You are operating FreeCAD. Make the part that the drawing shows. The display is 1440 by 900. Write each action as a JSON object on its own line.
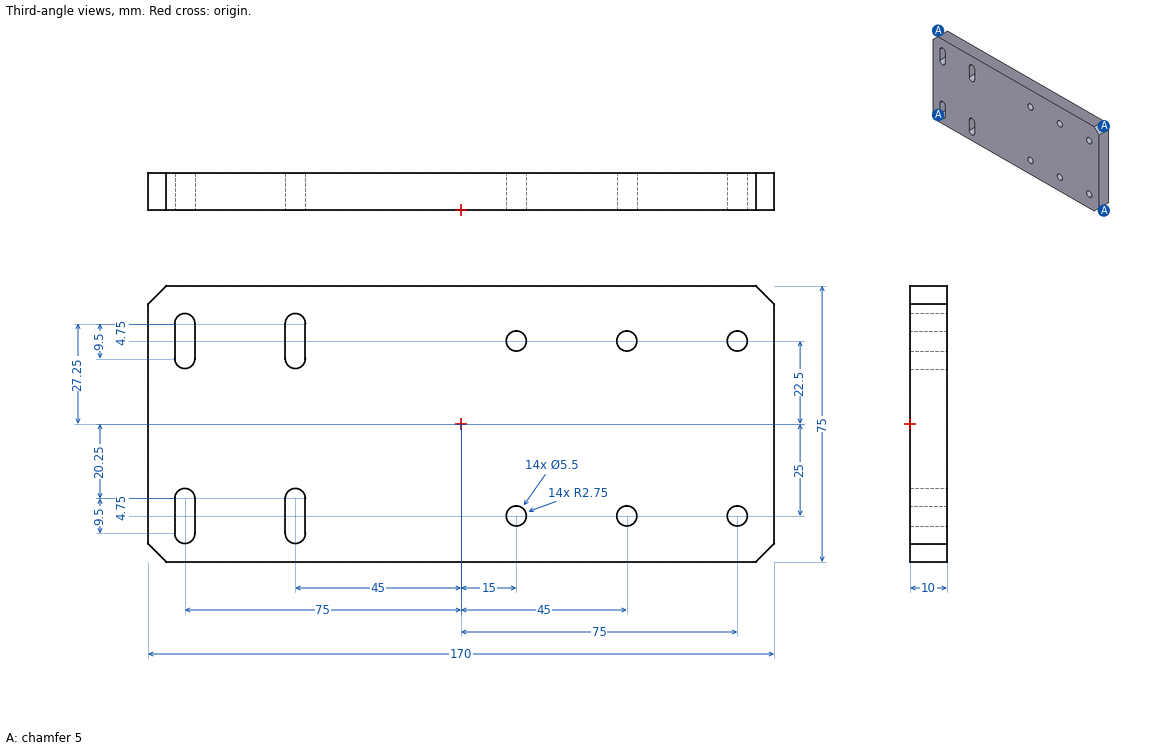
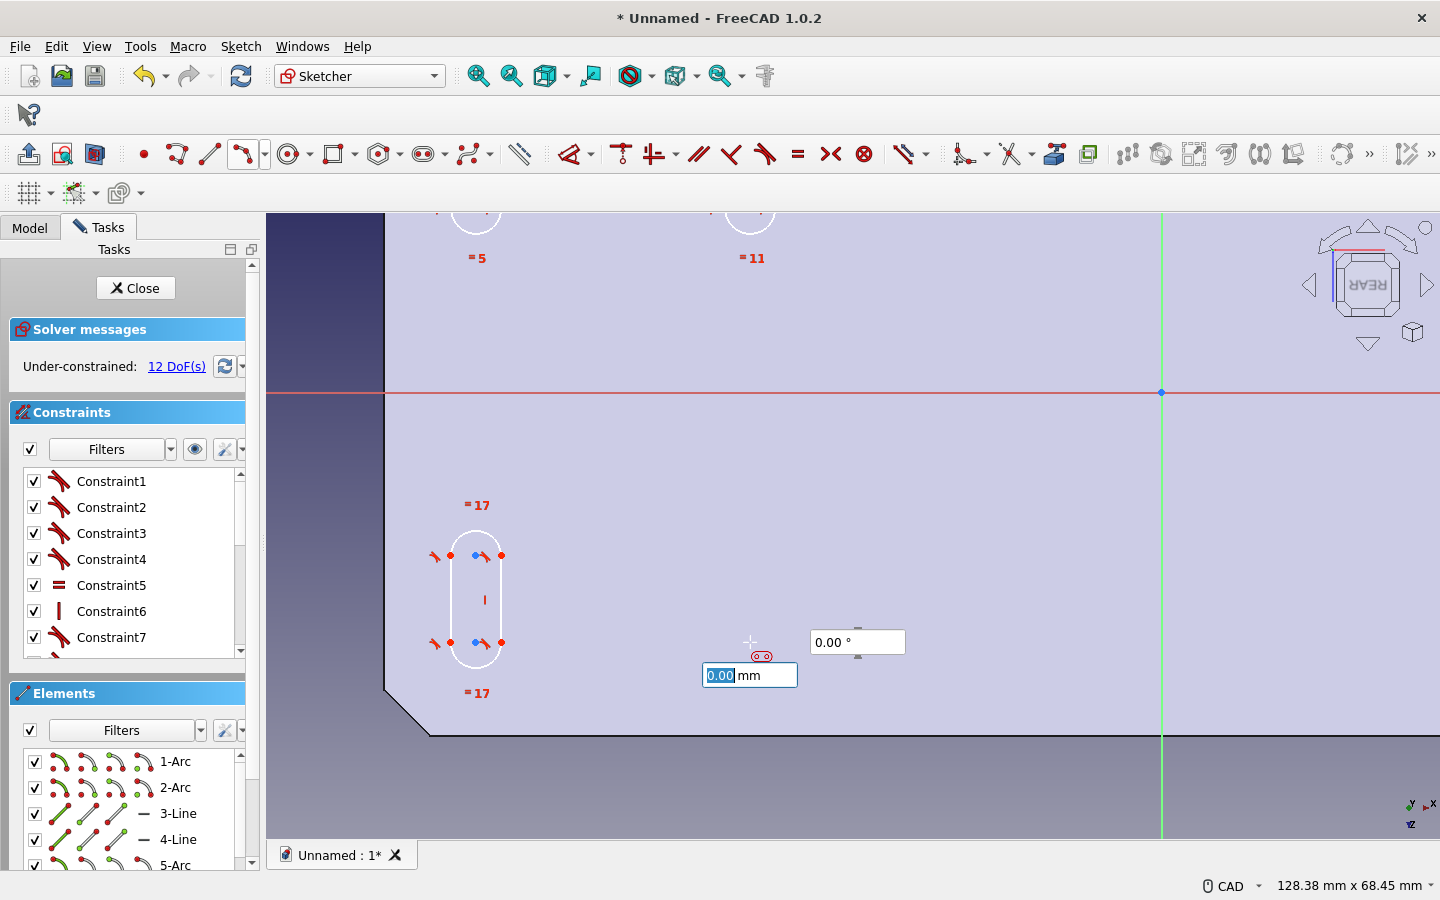
{"action": "left_click", "coordinate": [750, 555]}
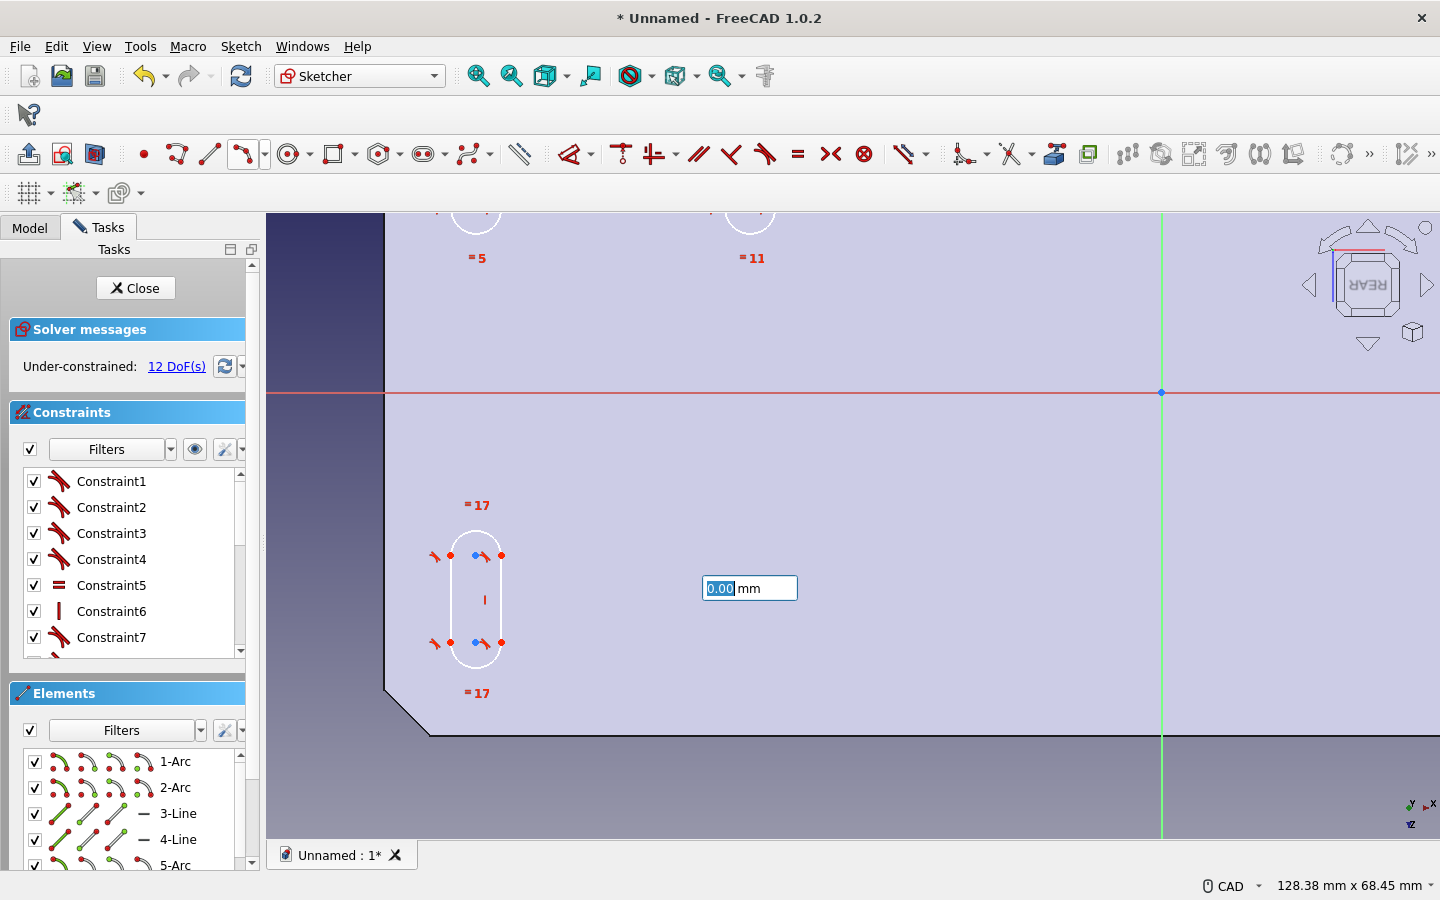
{"action": "left_click", "coordinate": [775, 599]}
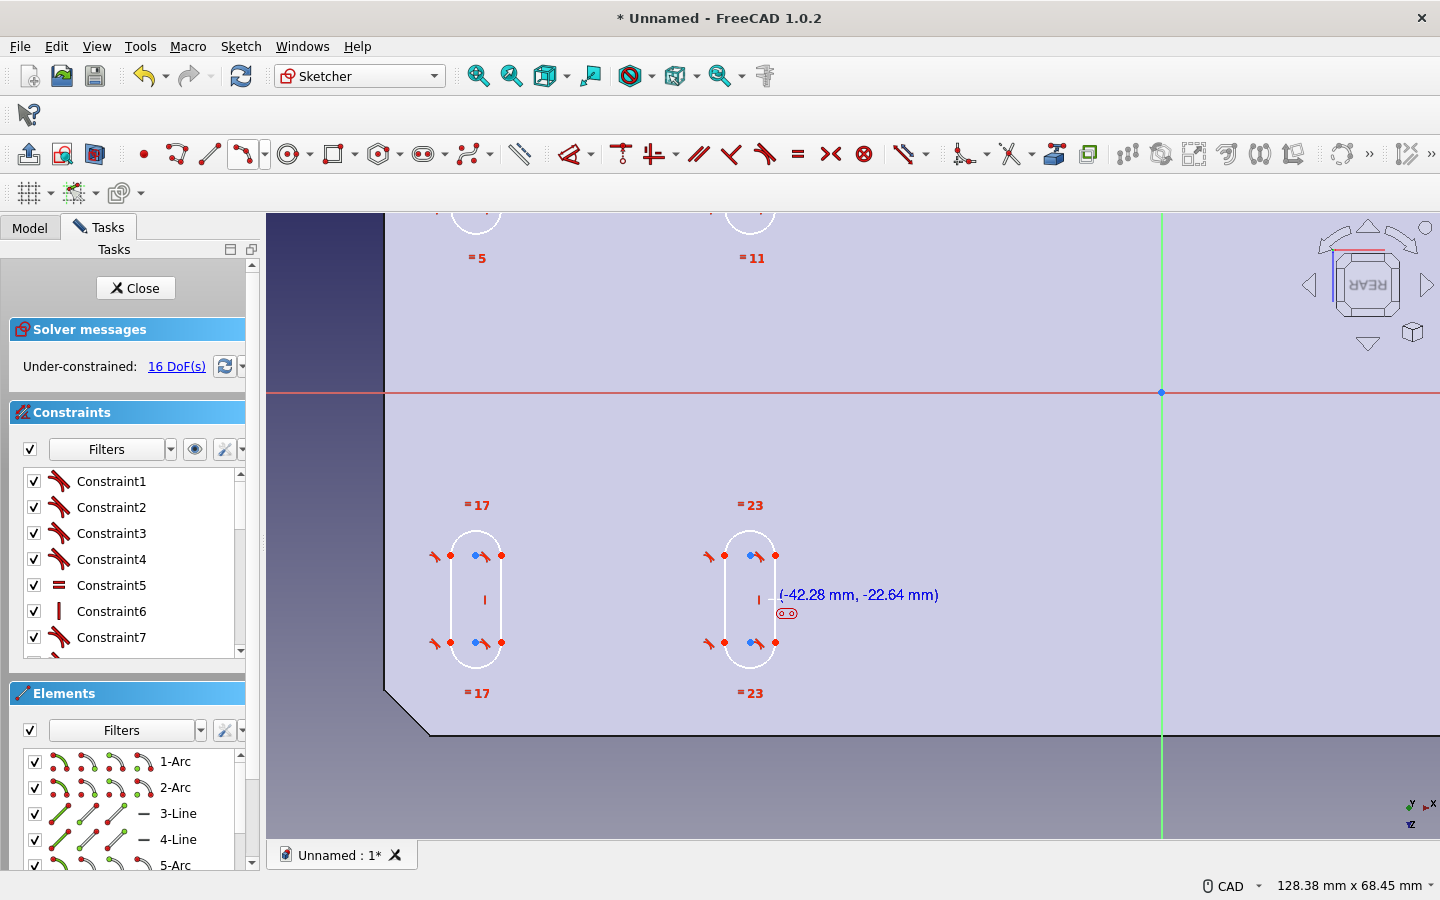
{"action": "key", "text": "g c"}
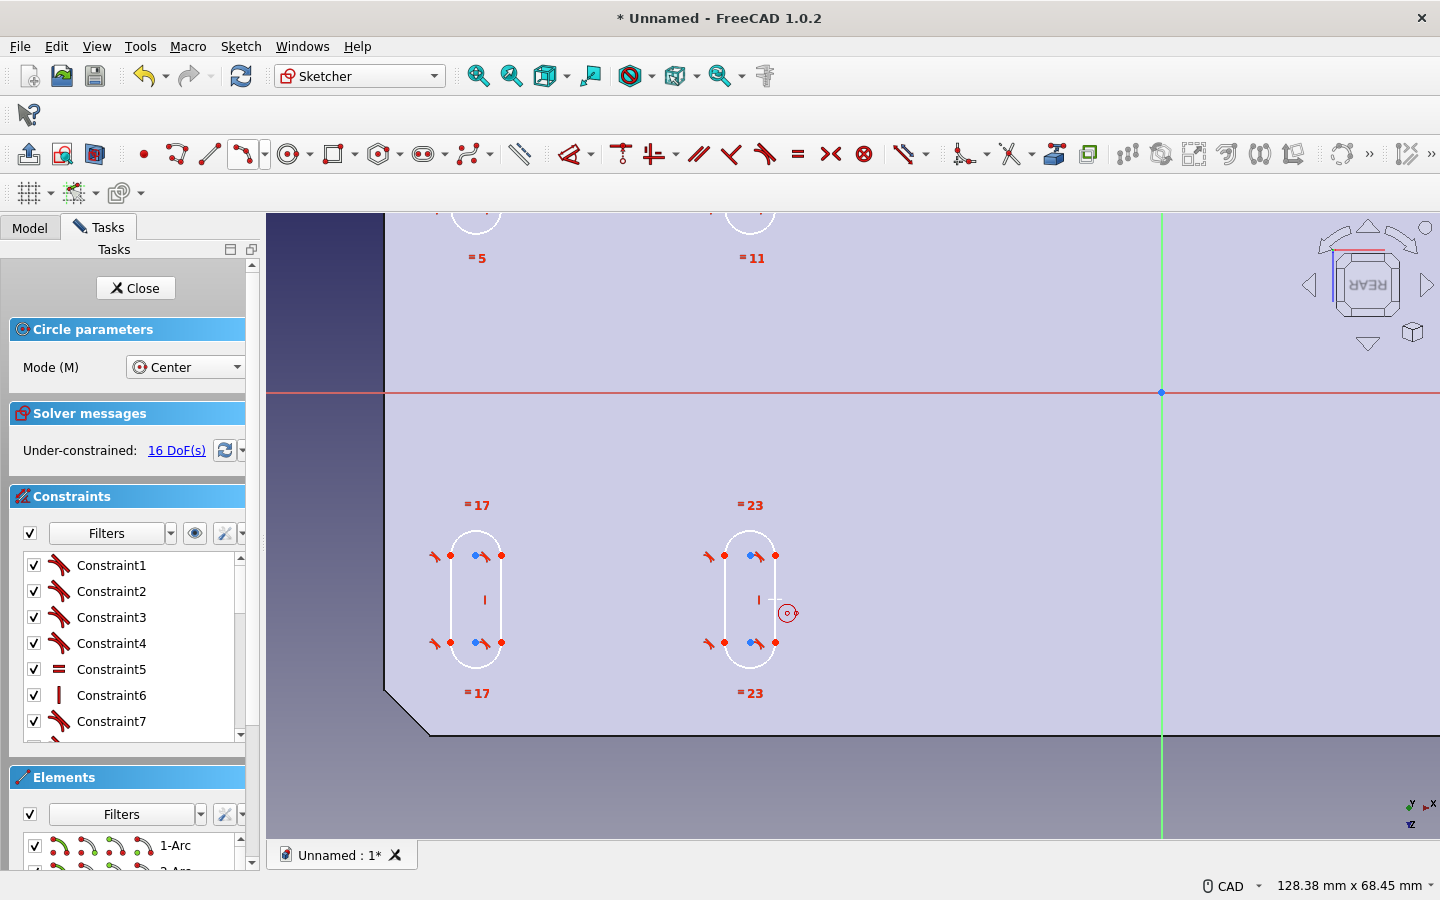
{"action": "scroll", "coordinate": [477, 644], "scroll_direction": "down", "scroll_amount": 4}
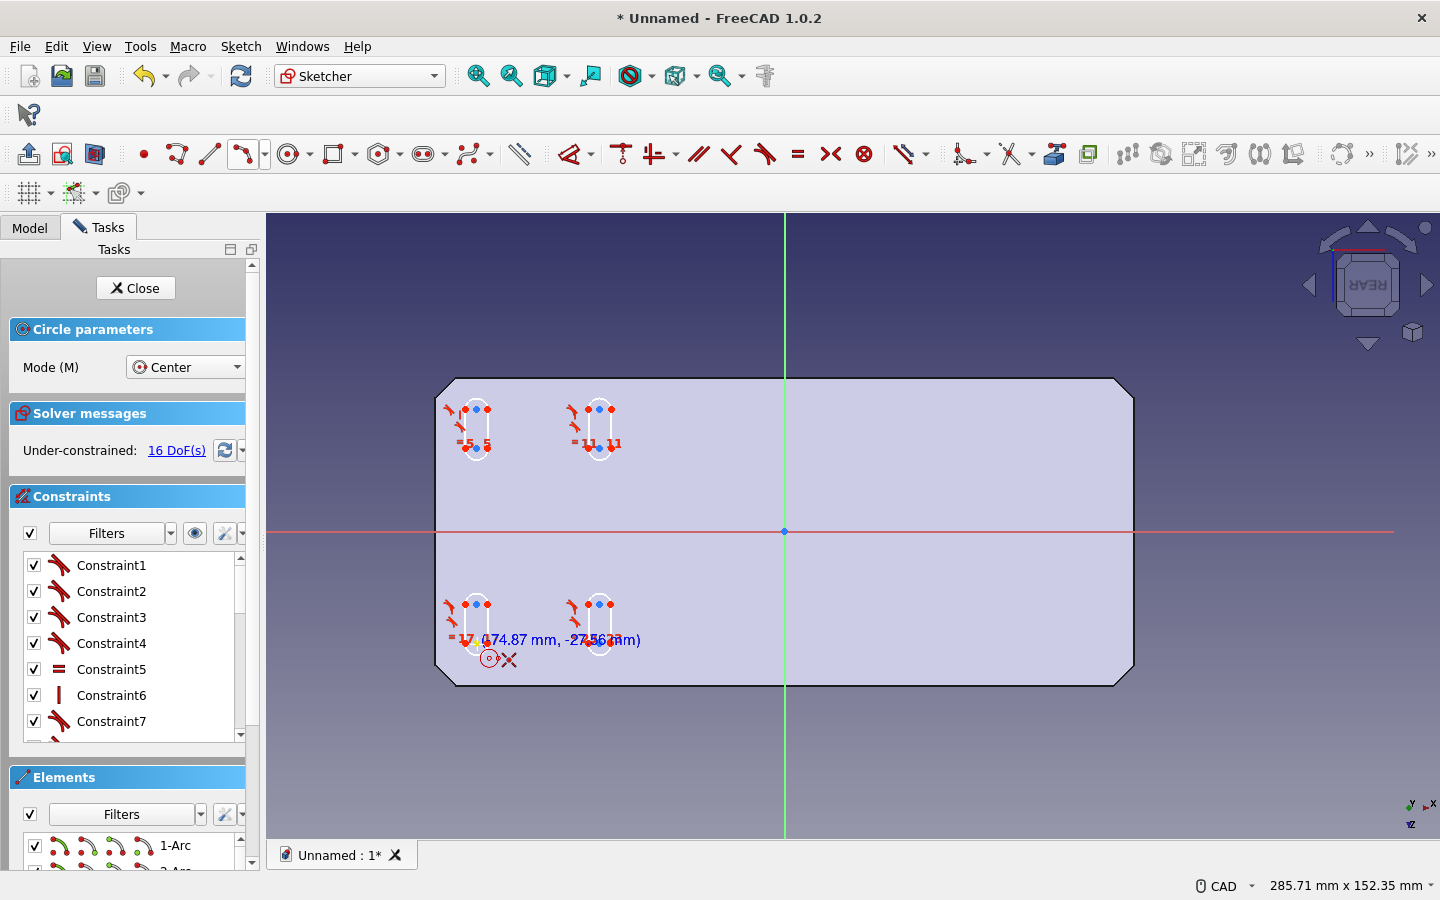
{"action": "scroll", "coordinate": [846, 429], "scroll_direction": "up", "scroll_amount": 4}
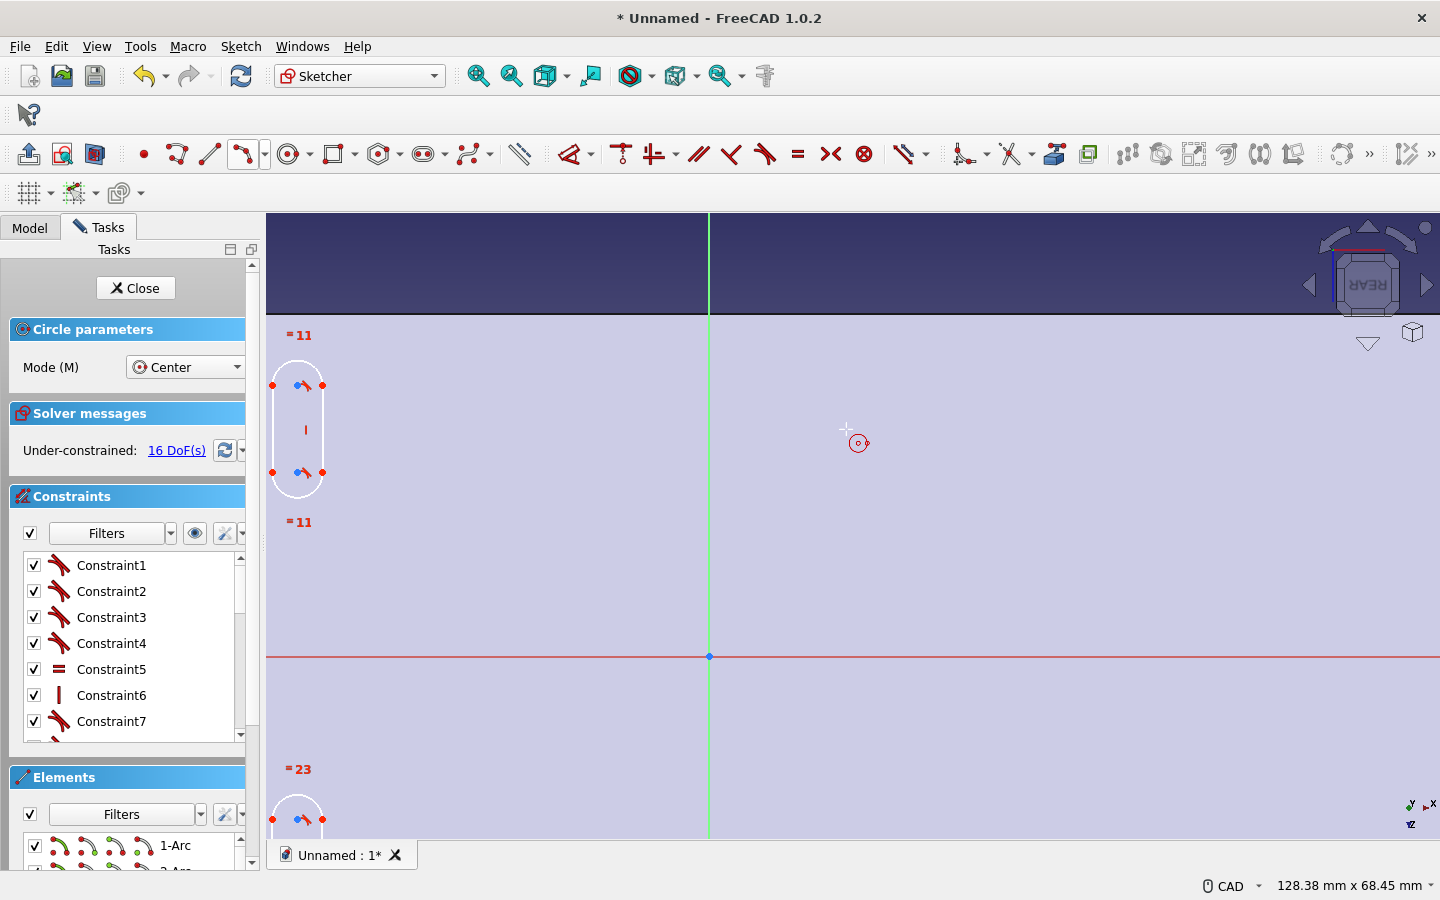
{"action": "left_click", "coordinate": [846, 428]}
{"action": "left_click", "coordinate": [864, 410]}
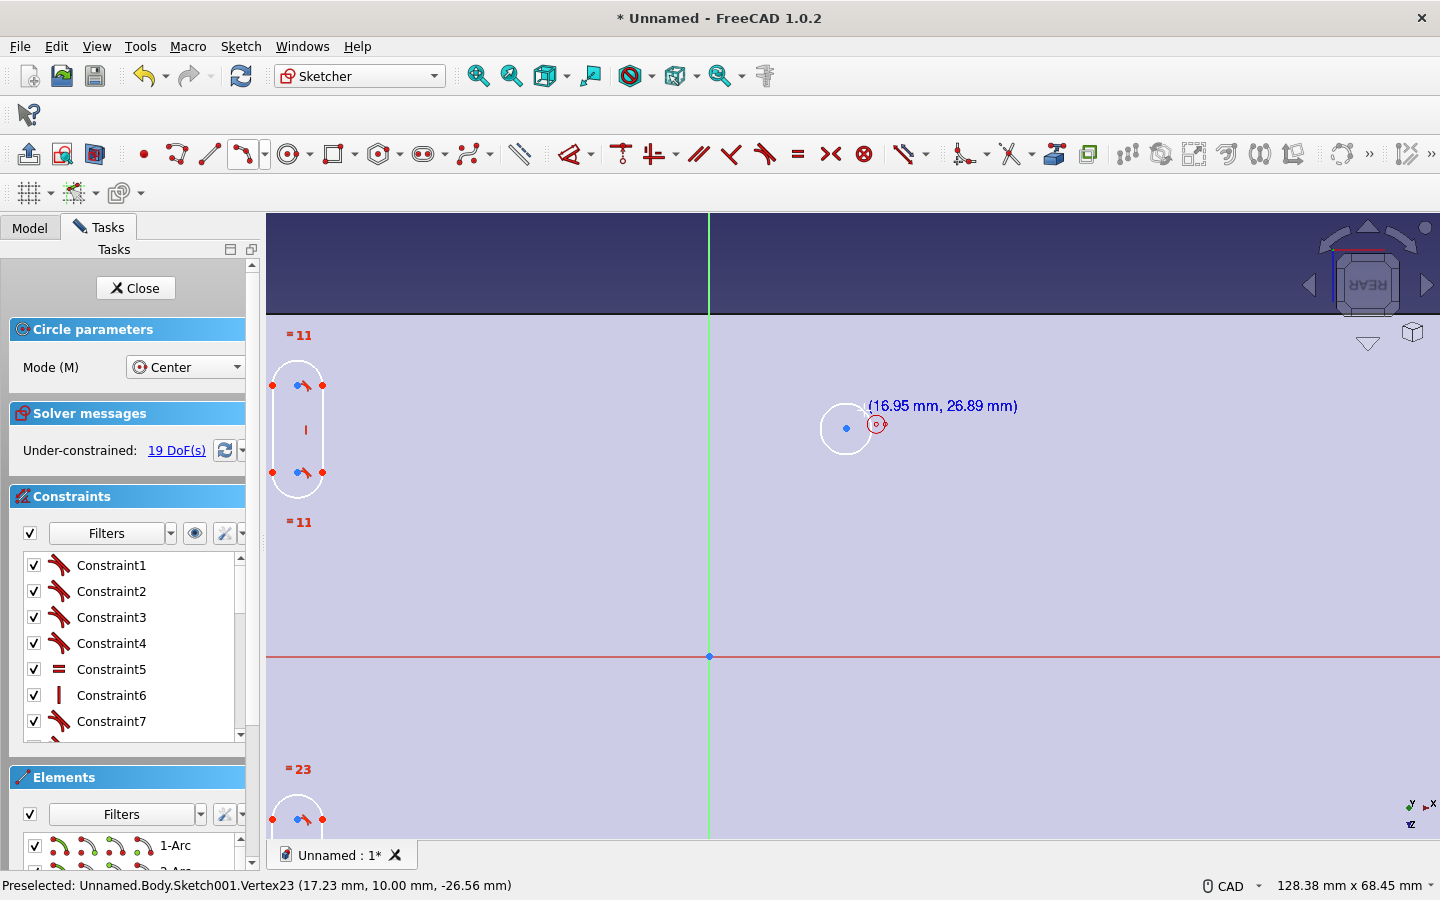
{"action": "left_click", "coordinate": [1121, 428]}
{"action": "left_click", "coordinate": [1138, 410]}